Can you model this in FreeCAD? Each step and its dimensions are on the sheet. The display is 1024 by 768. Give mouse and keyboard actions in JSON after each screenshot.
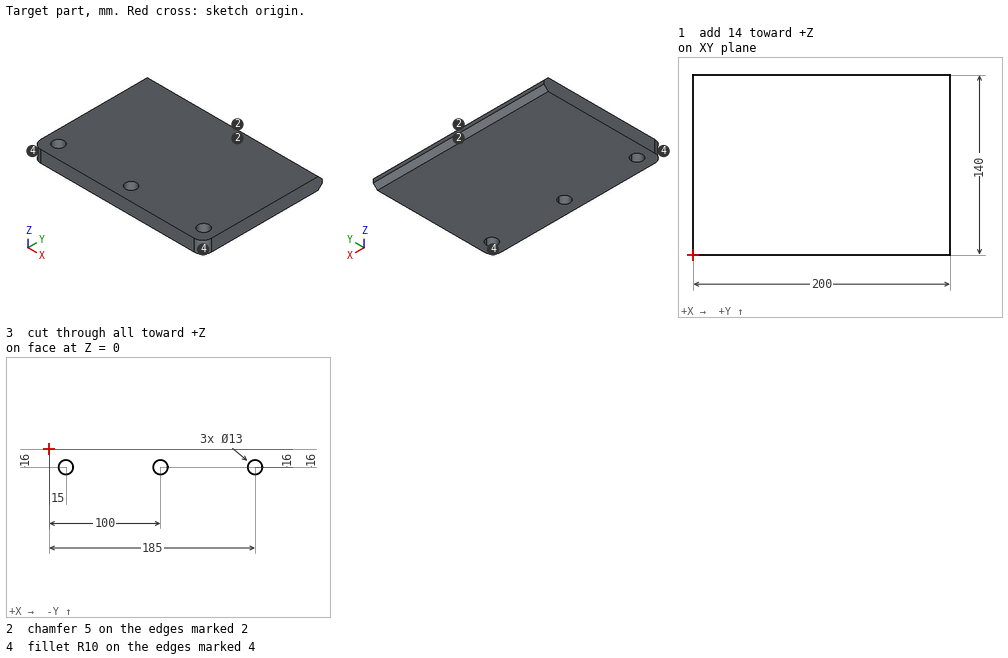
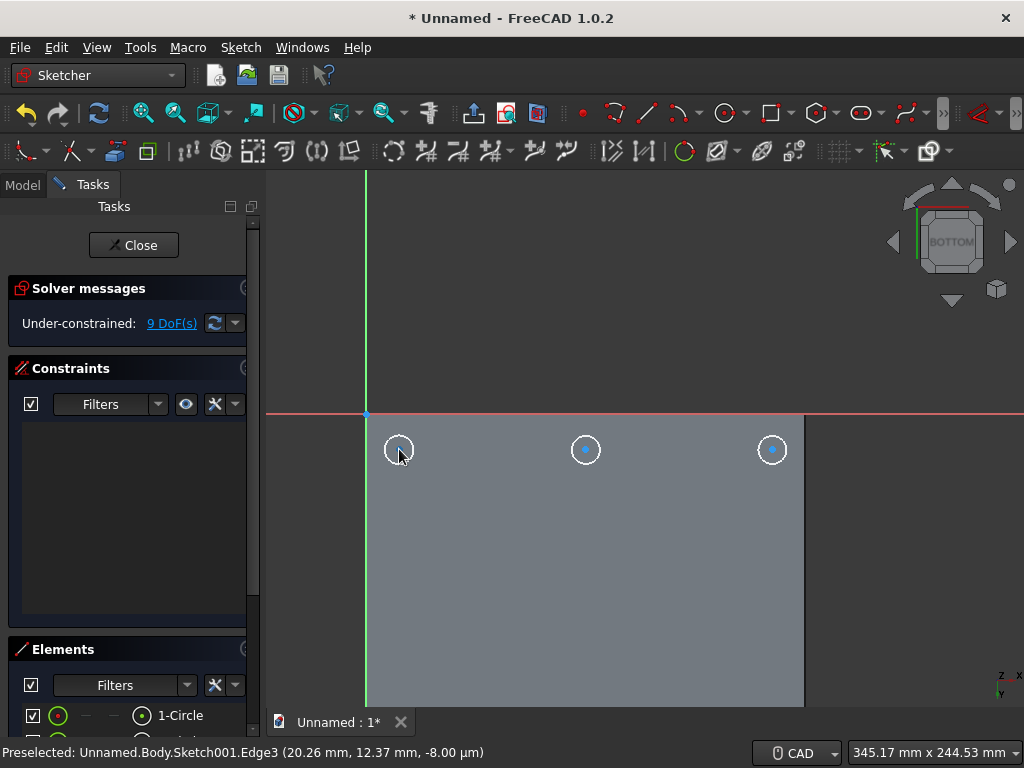
{"action": "left_click", "coordinate": [782, 440]}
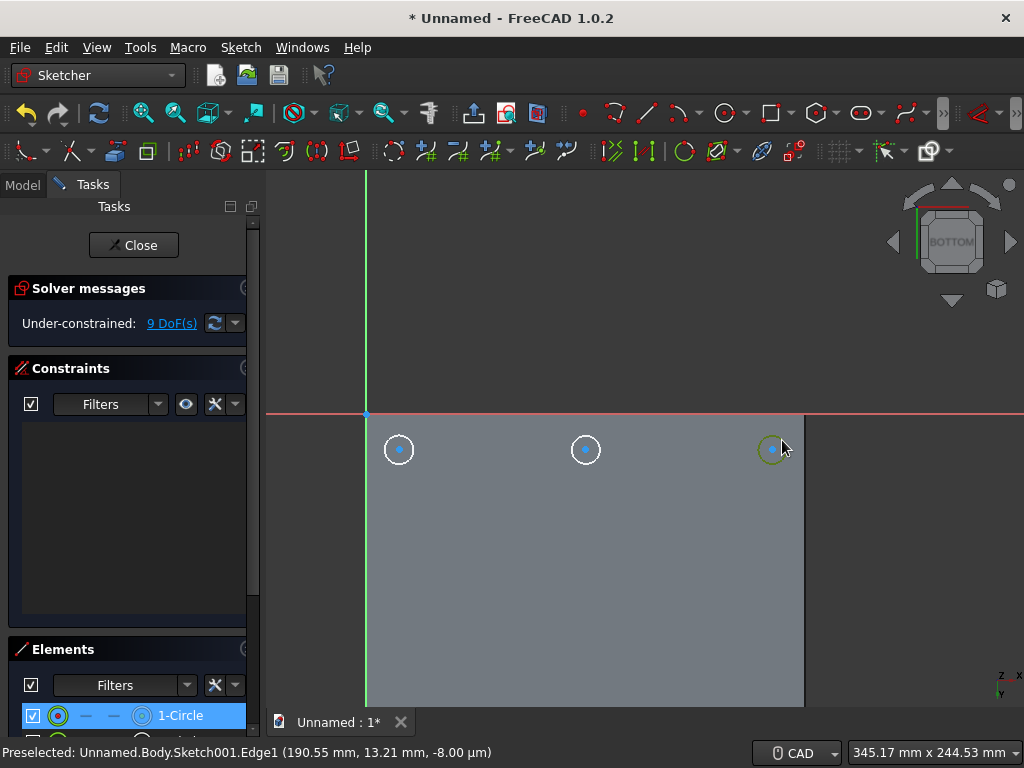
{"action": "left_click", "coordinate": [596, 440]}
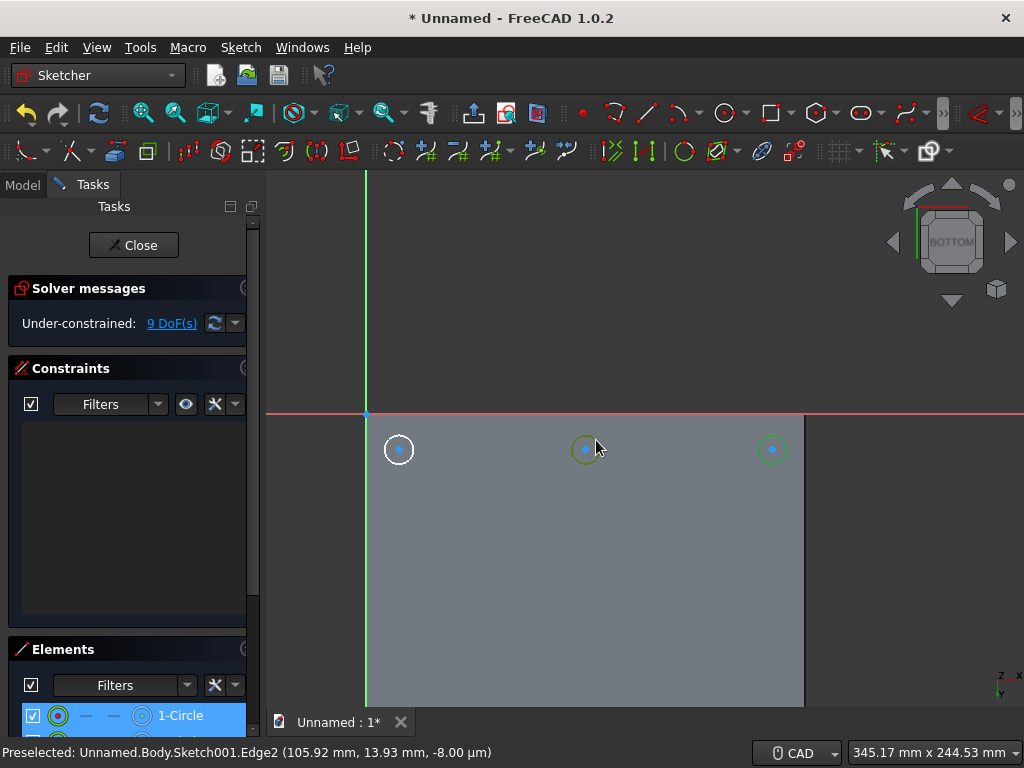
{"action": "left_click", "coordinate": [409, 440]}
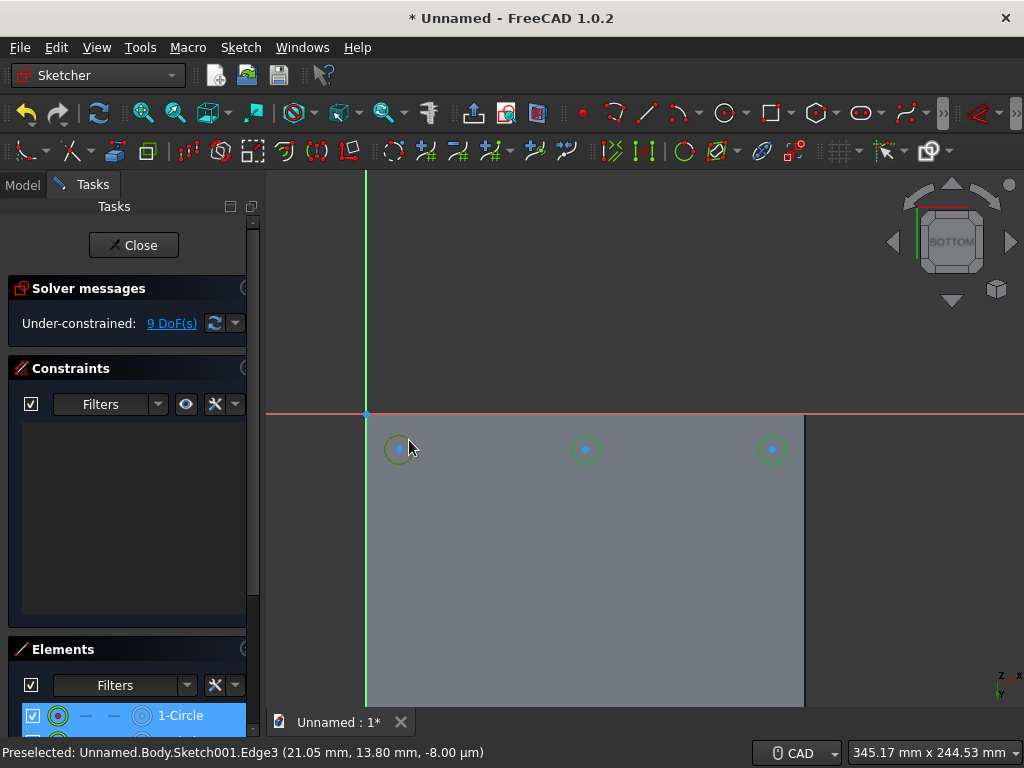
{"action": "key", "text": "e"}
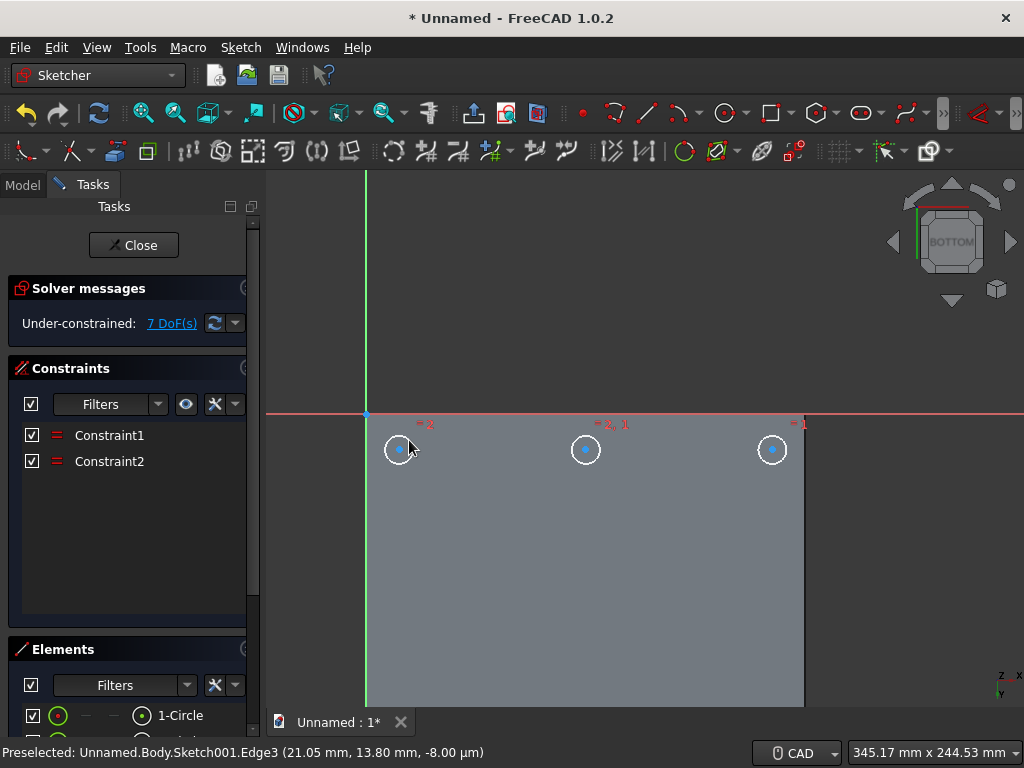
{"action": "left_click", "coordinate": [978, 114]}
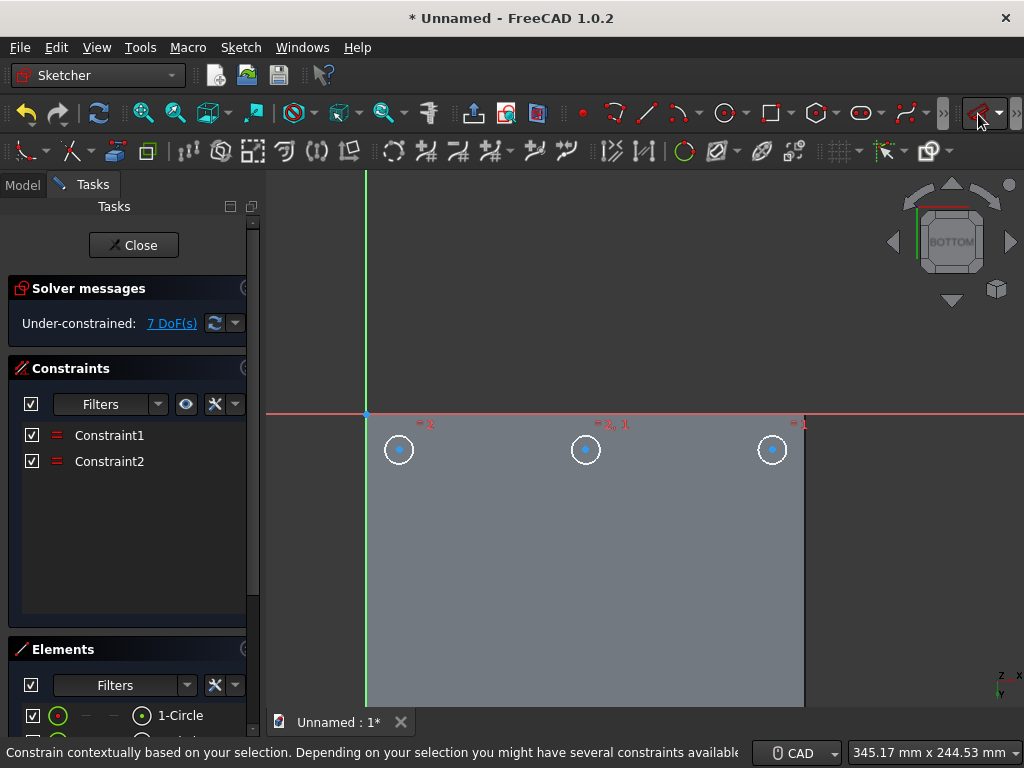
{"action": "scroll", "coordinate": [782, 440], "scroll_direction": "up", "scroll_amount": 2}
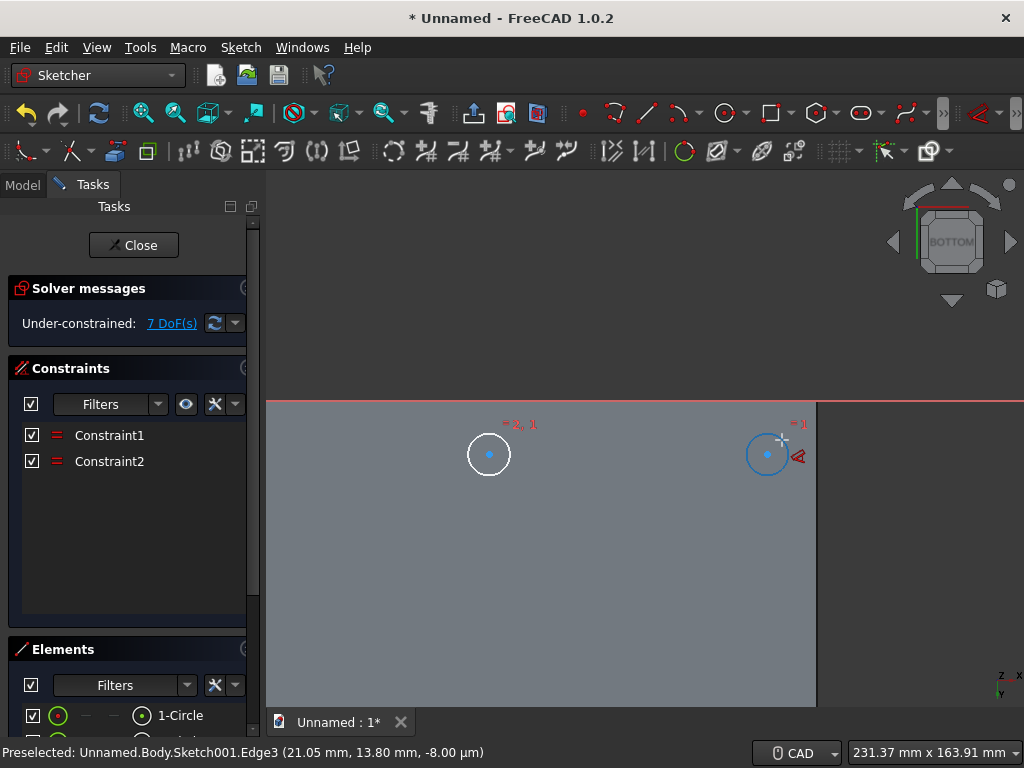
{"action": "left_click", "coordinate": [782, 440]}
{"action": "left_click", "coordinate": [805, 417]}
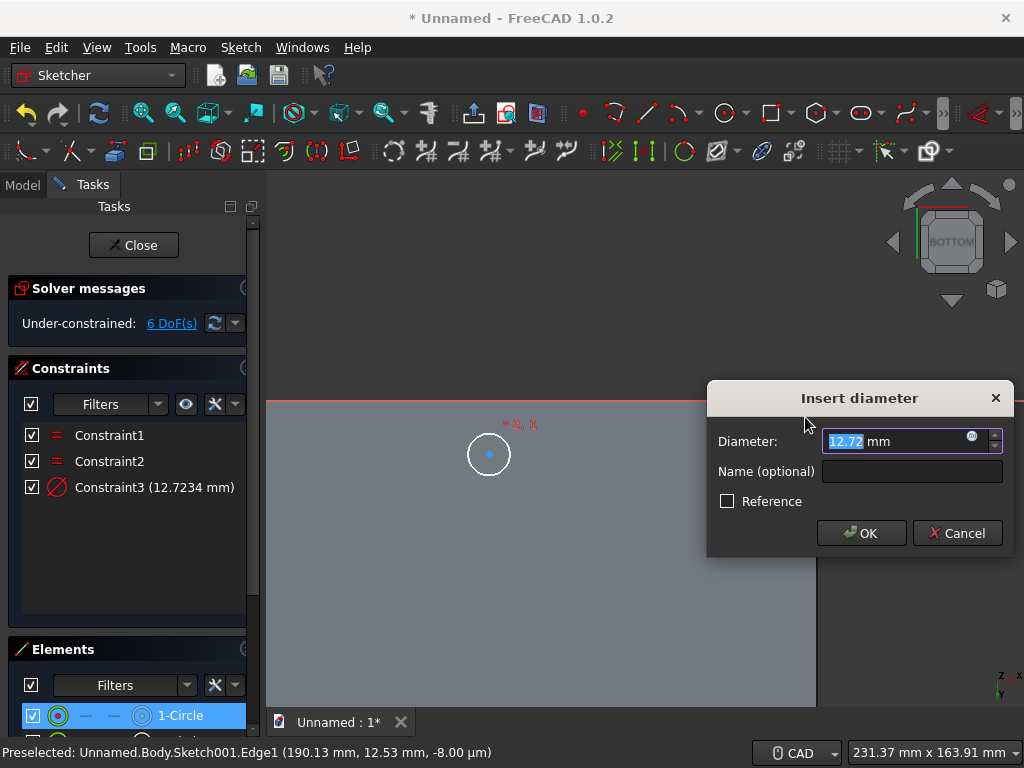
{"action": "type", "text": "13"}
{"action": "key", "text": "Return"}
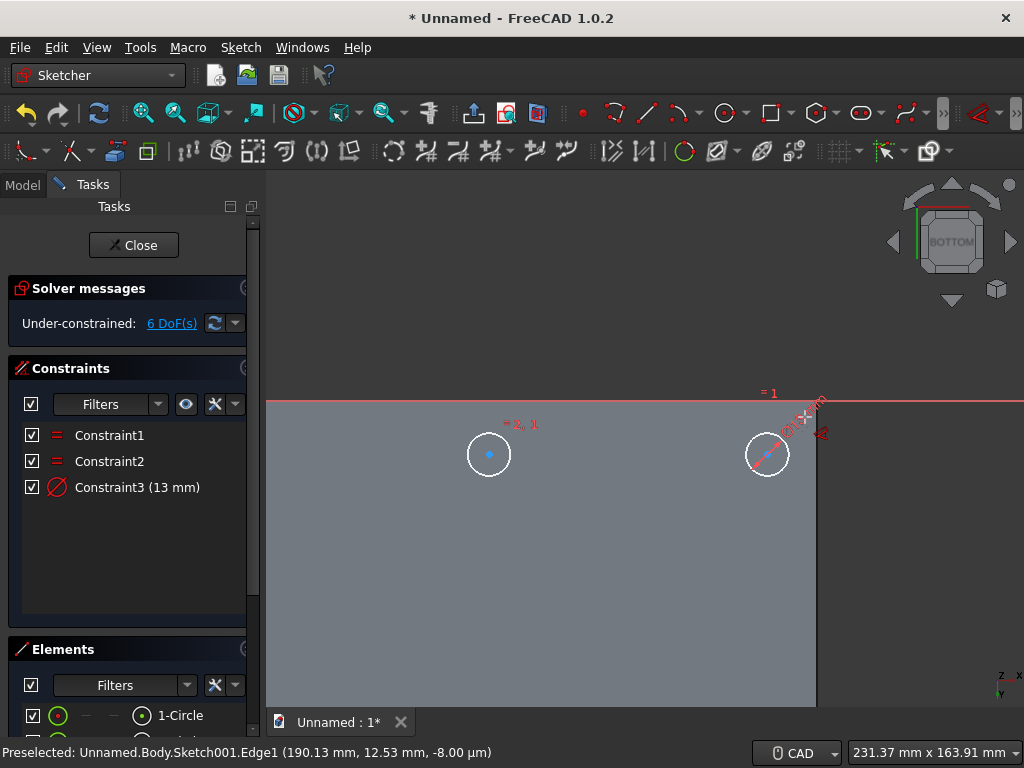
{"action": "left_click", "coordinate": [767, 455]}
{"action": "left_click", "coordinate": [801, 440]}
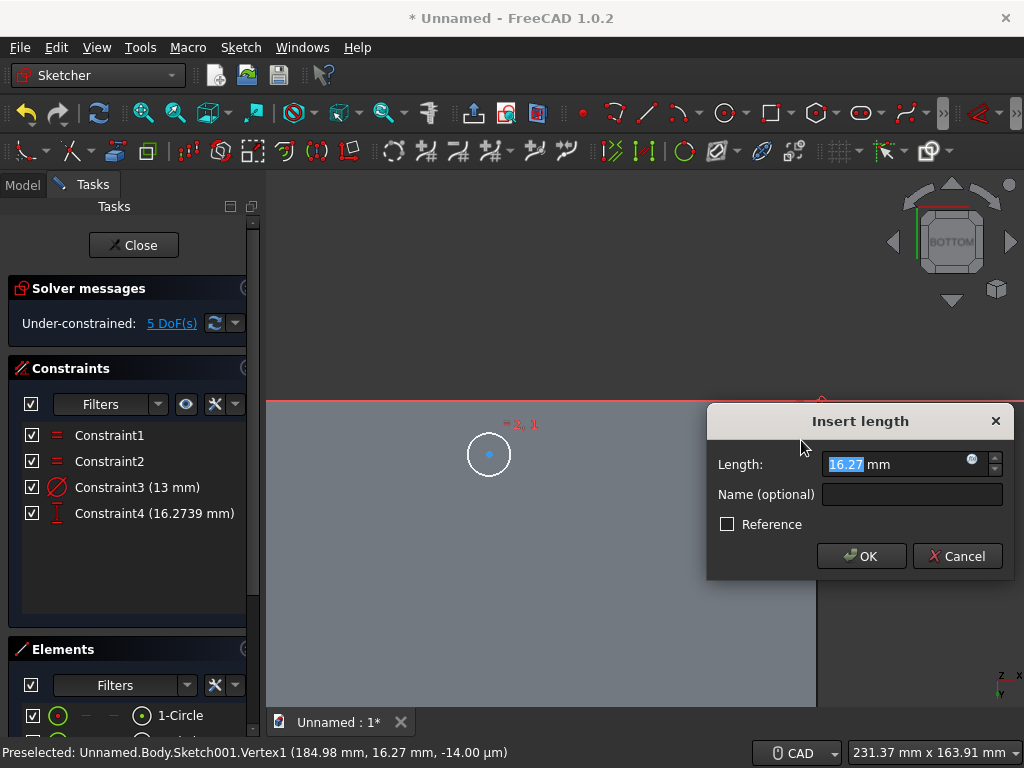
{"action": "type", "text": "16"}
{"action": "key", "text": "Return"}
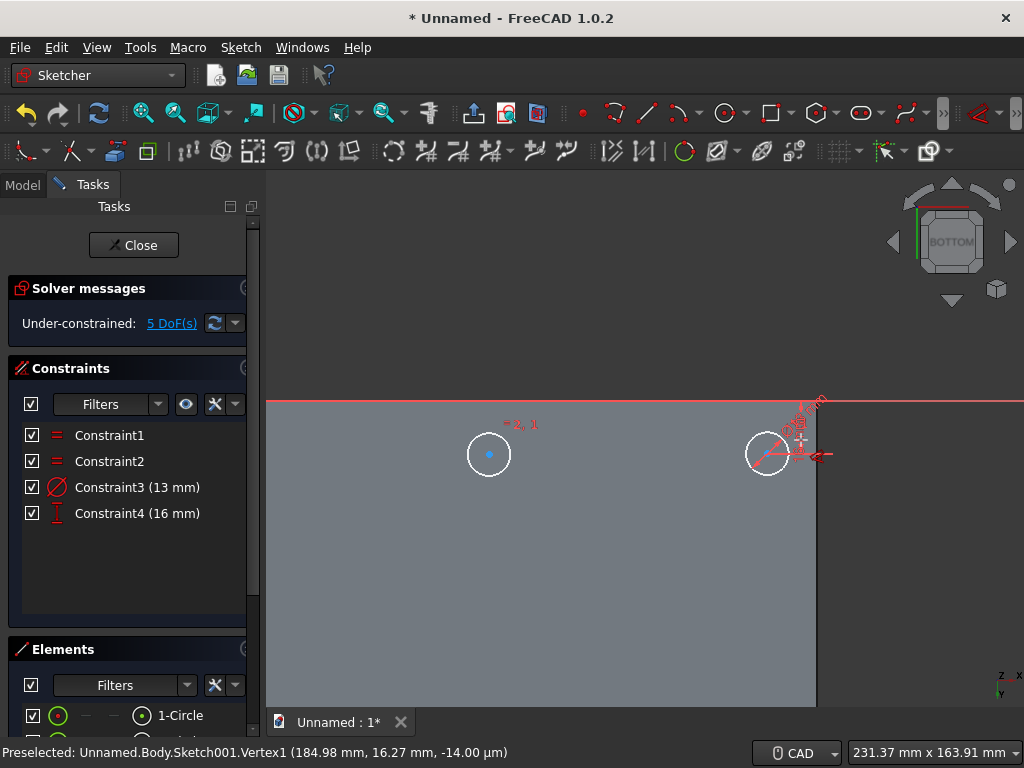
{"action": "left_click", "coordinate": [489, 455]}
{"action": "left_click", "coordinate": [523, 428]}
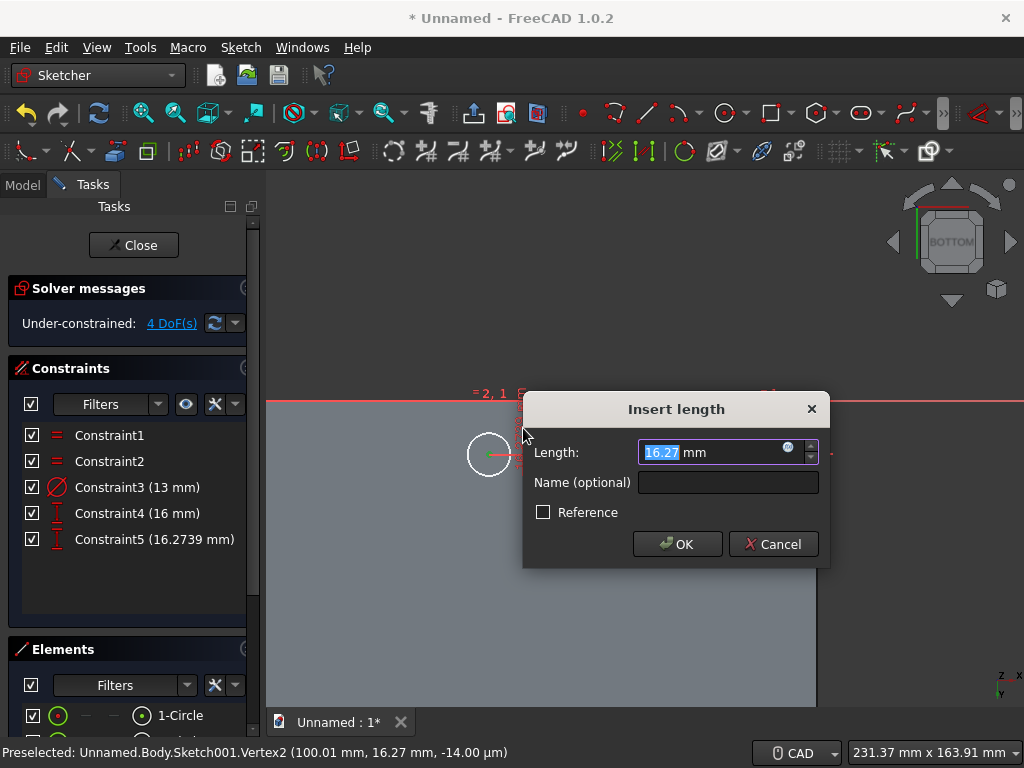
{"action": "type", "text": "16"}
{"action": "key", "text": "Return"}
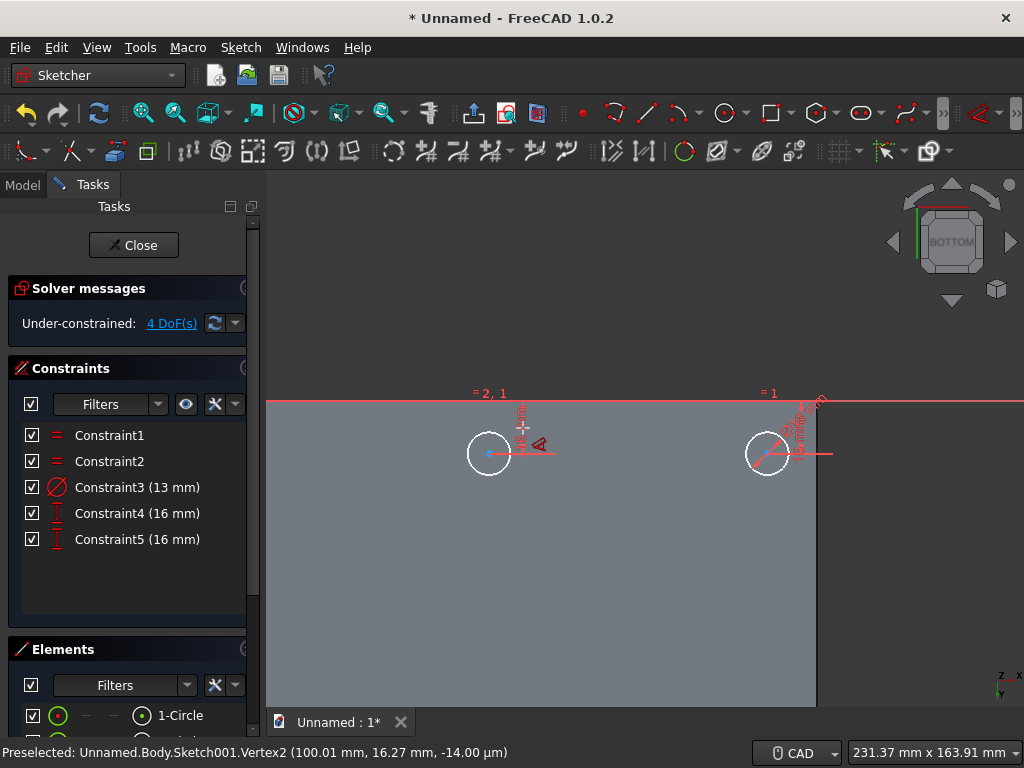
{"action": "scroll", "coordinate": [783, 439], "scroll_direction": "down", "scroll_amount": 2}